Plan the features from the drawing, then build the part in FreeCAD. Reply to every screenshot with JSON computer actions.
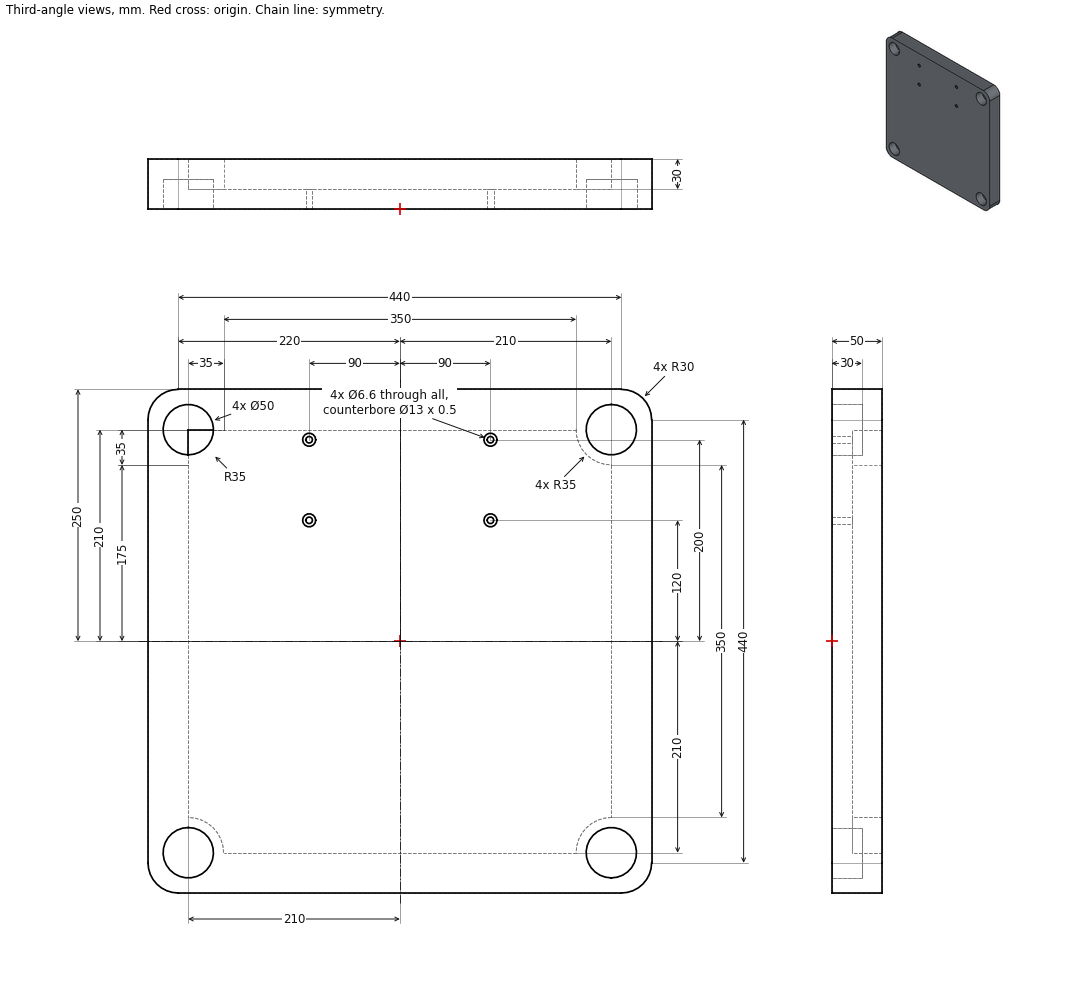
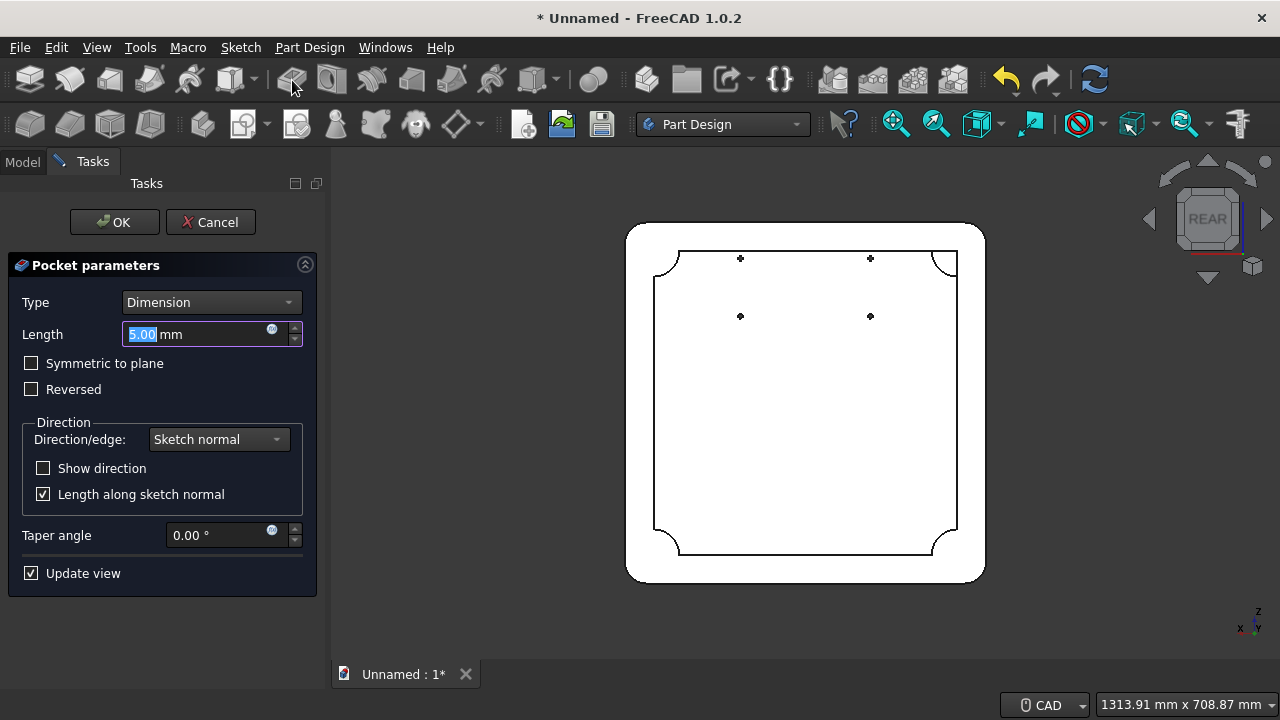
{"action": "type", "text": "30"}
{"action": "key", "text": "Tab"}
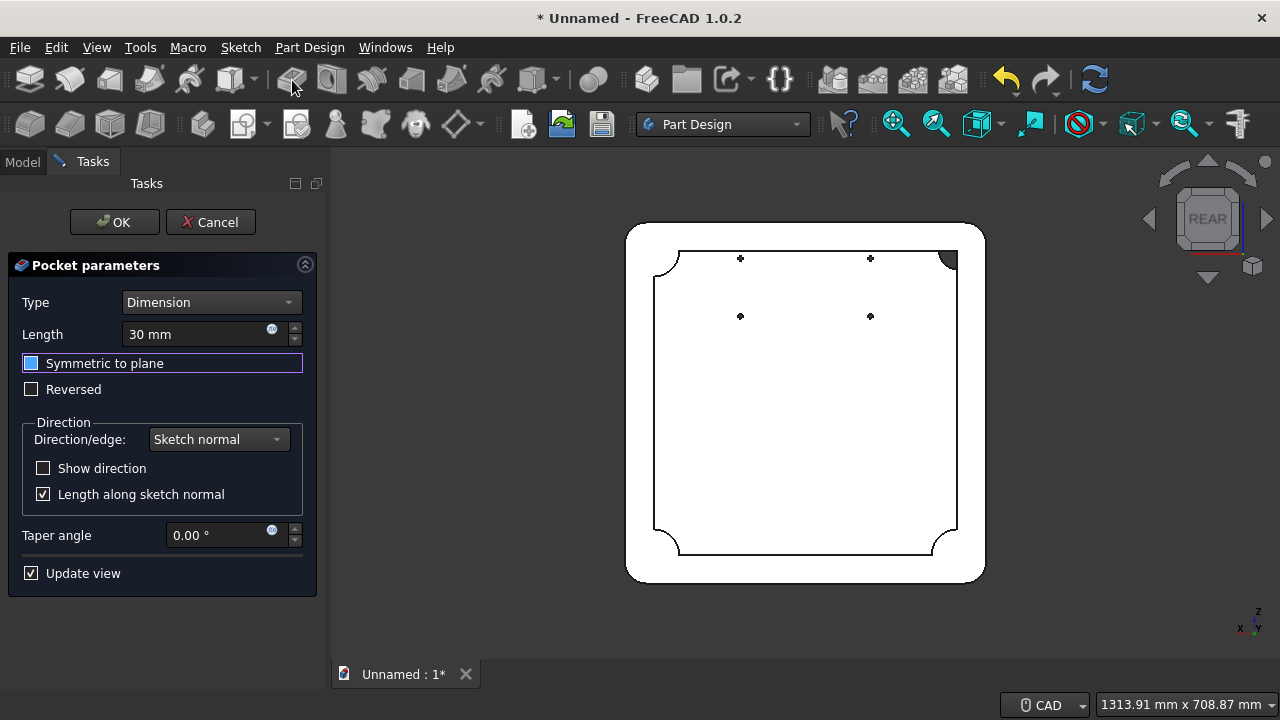
{"action": "left_click", "coordinate": [115, 222]}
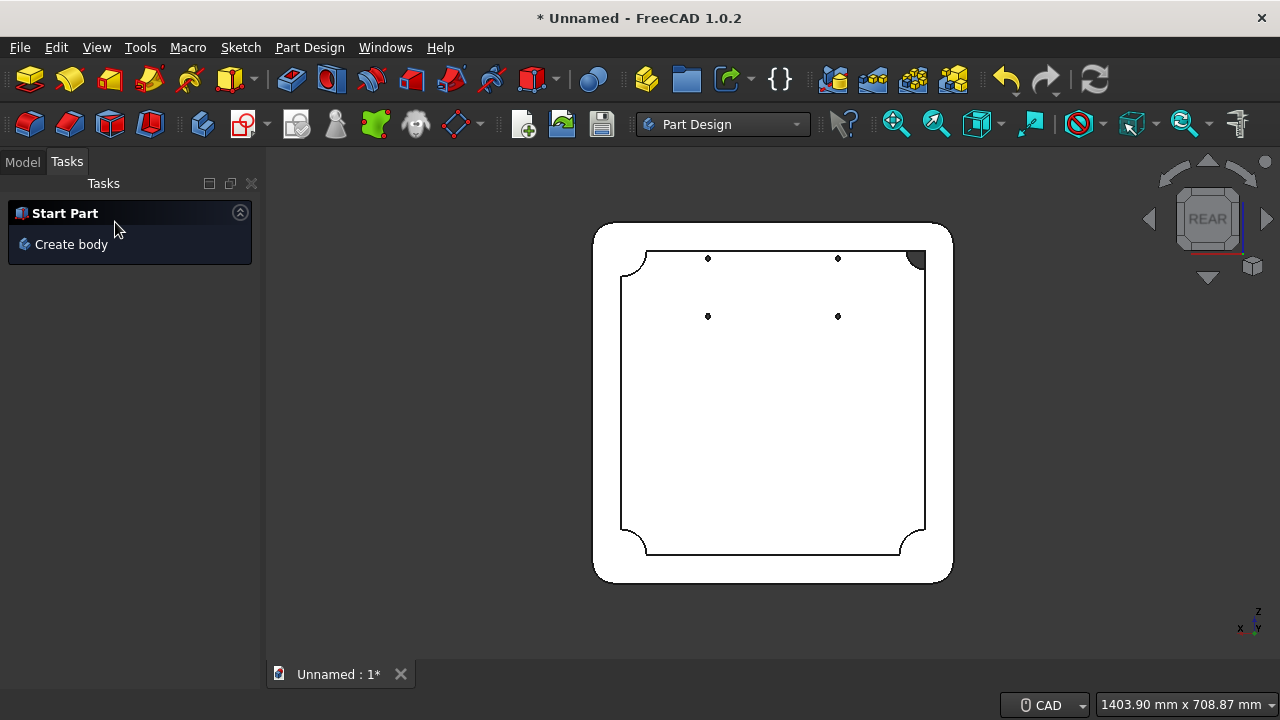
{"action": "key", "text": "0"}